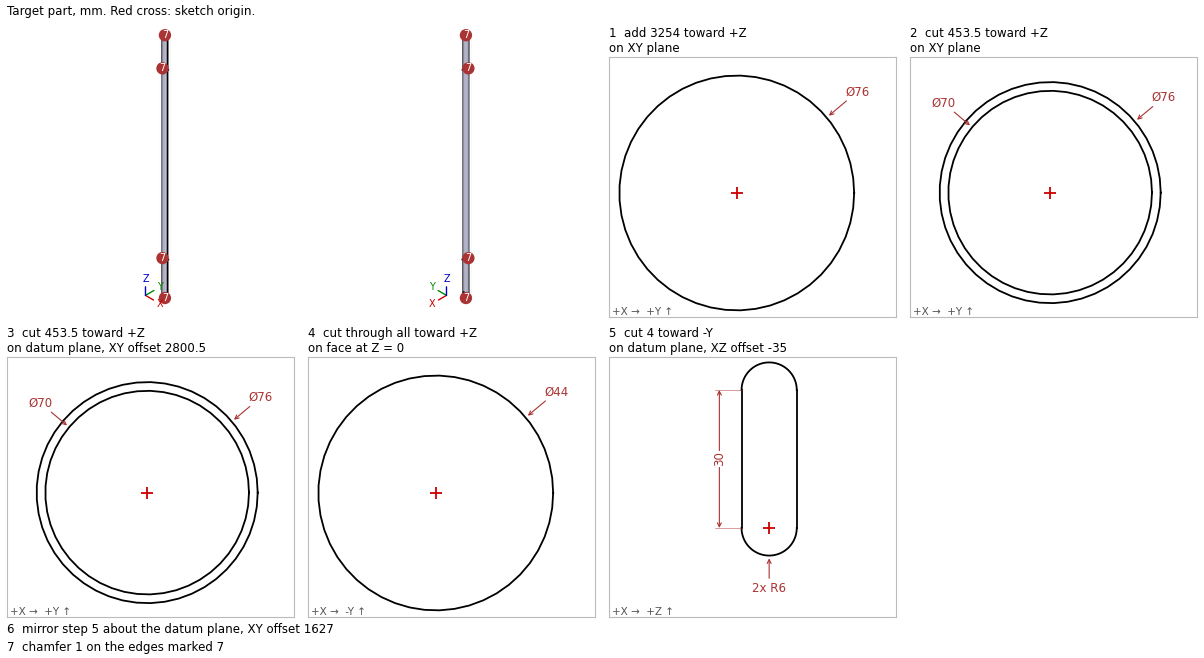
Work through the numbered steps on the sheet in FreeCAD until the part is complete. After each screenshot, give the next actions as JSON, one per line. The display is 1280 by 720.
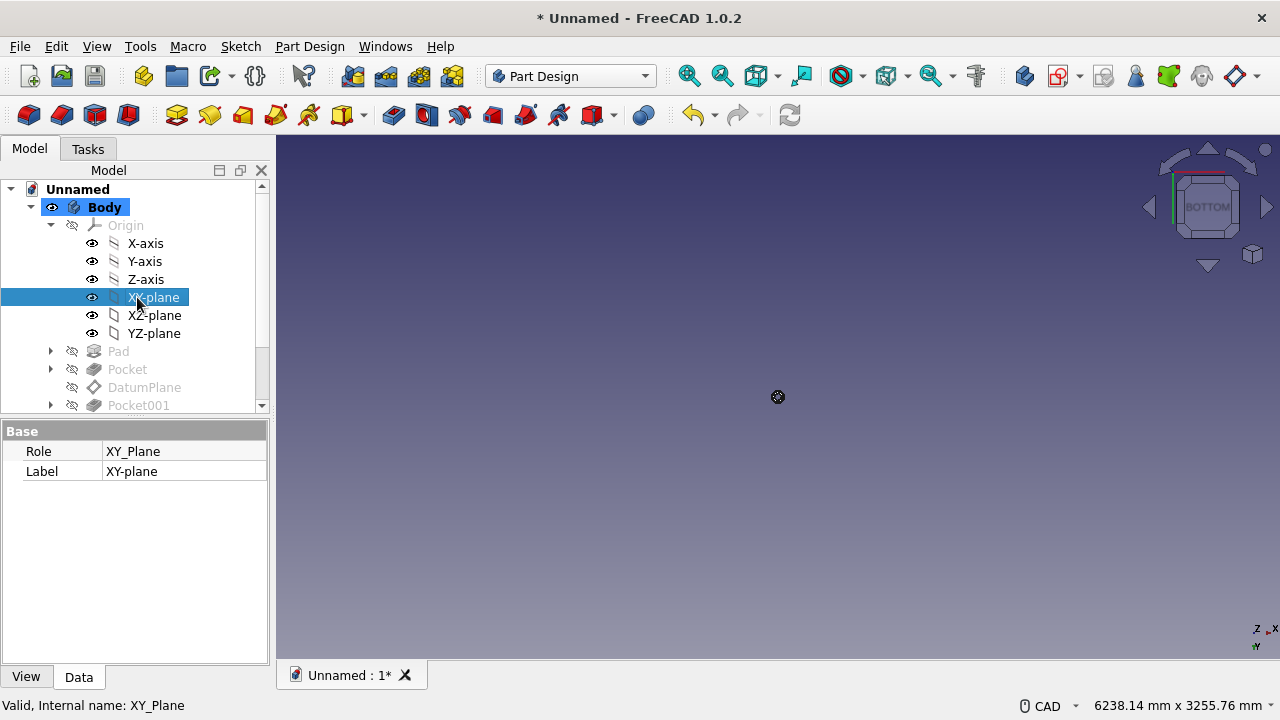
{"action": "left_click", "coordinate": [1234, 76]}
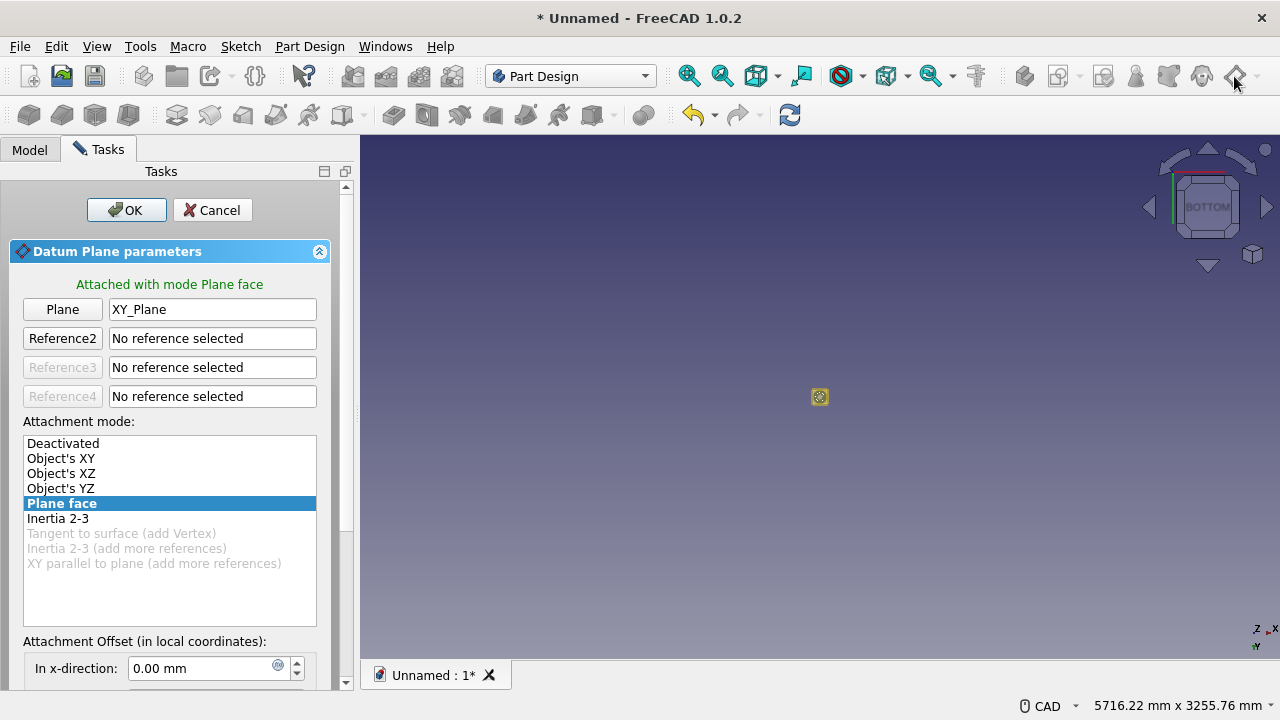
{"action": "scroll", "coordinate": [346, 436], "scroll_direction": "down", "scroll_amount": 2}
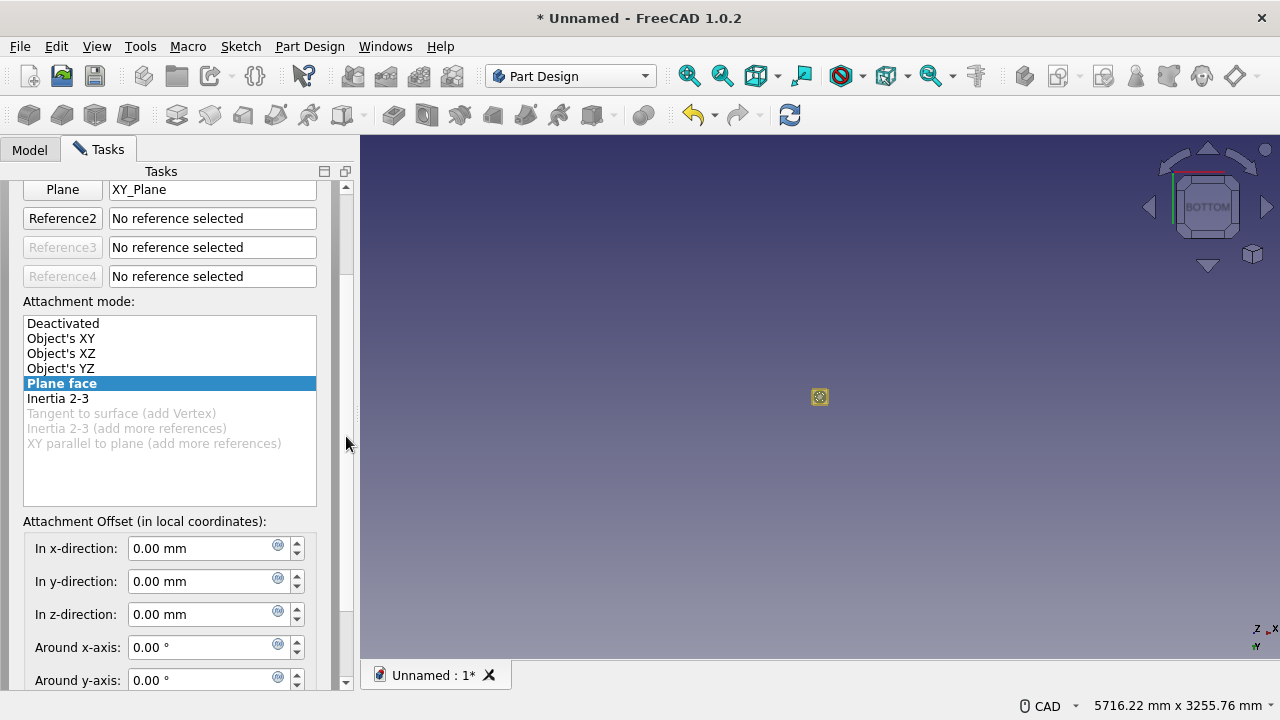
{"action": "triple_click", "coordinate": [210, 614]}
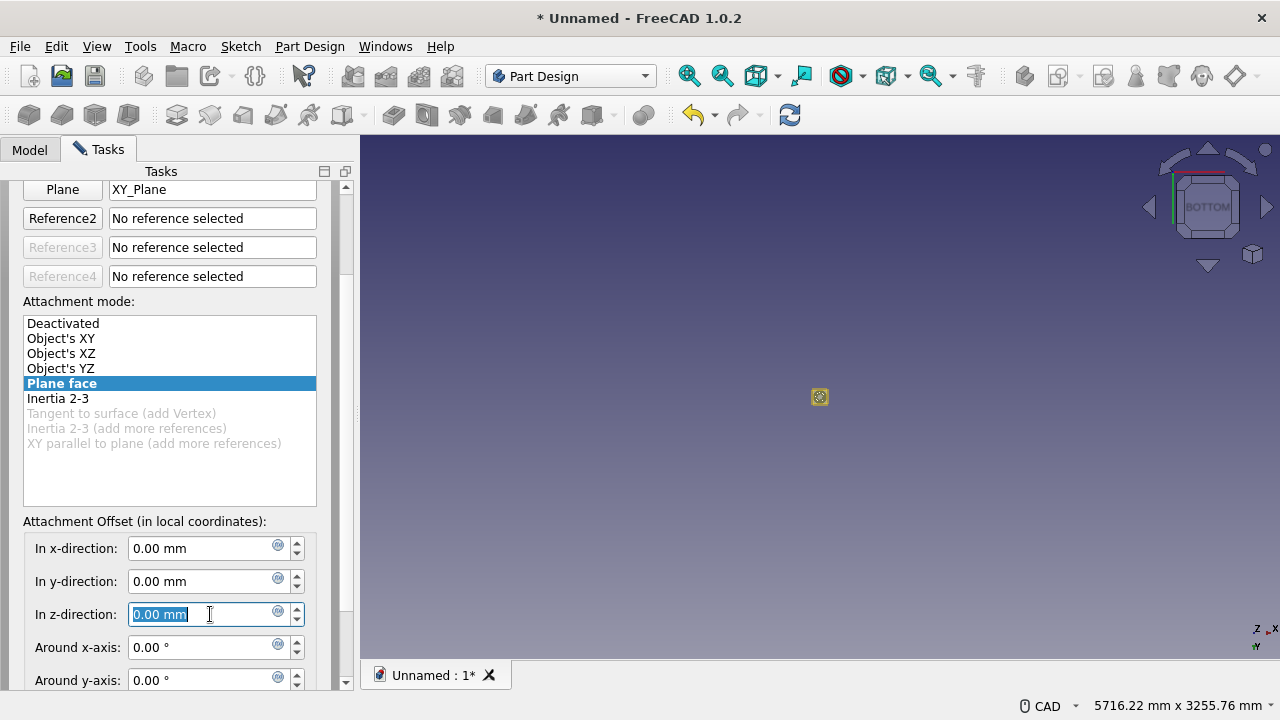
{"action": "type", "text": "1627"}
{"action": "key", "text": "Tab"}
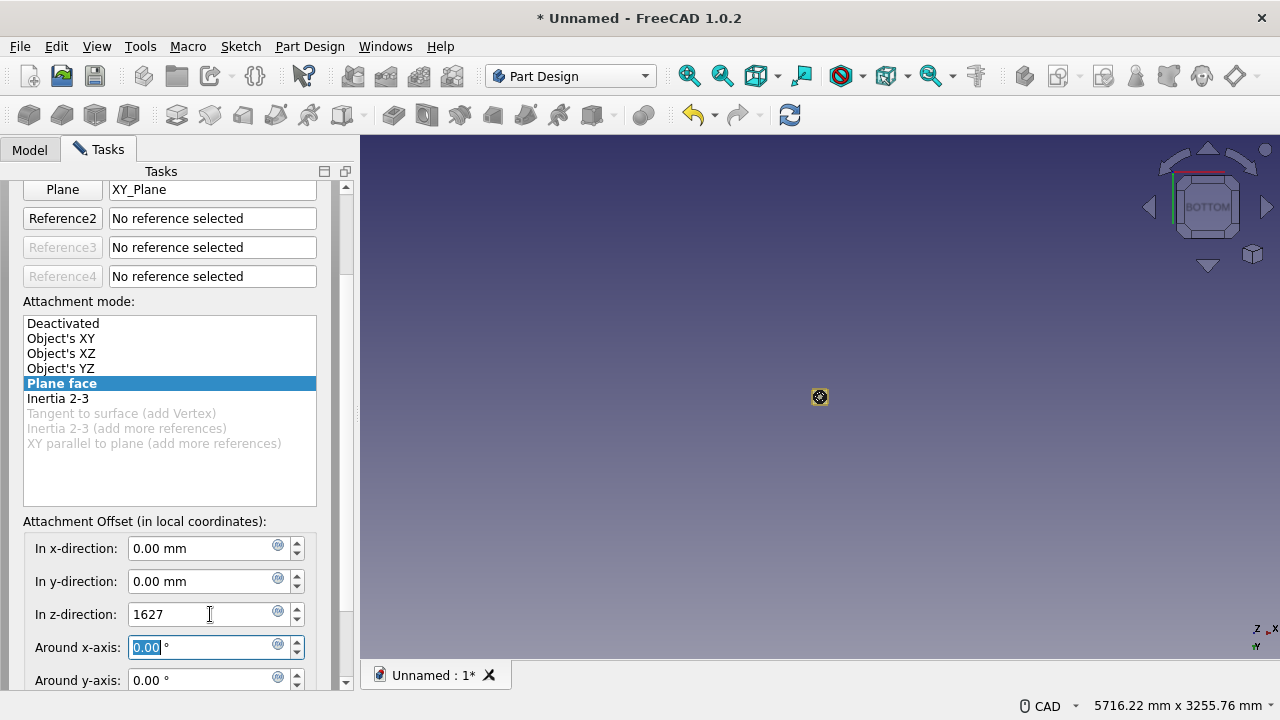
{"action": "scroll", "coordinate": [346, 436], "scroll_direction": "up", "scroll_amount": 3}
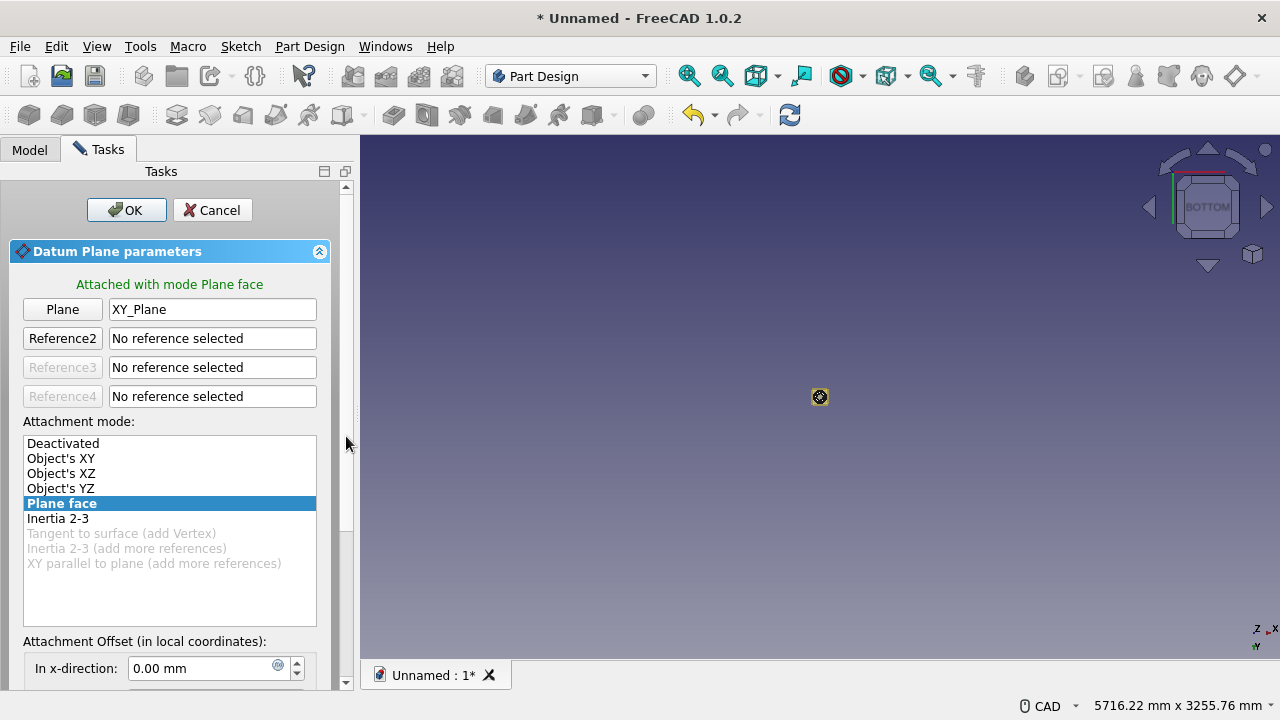
{"action": "left_click", "coordinate": [127, 210]}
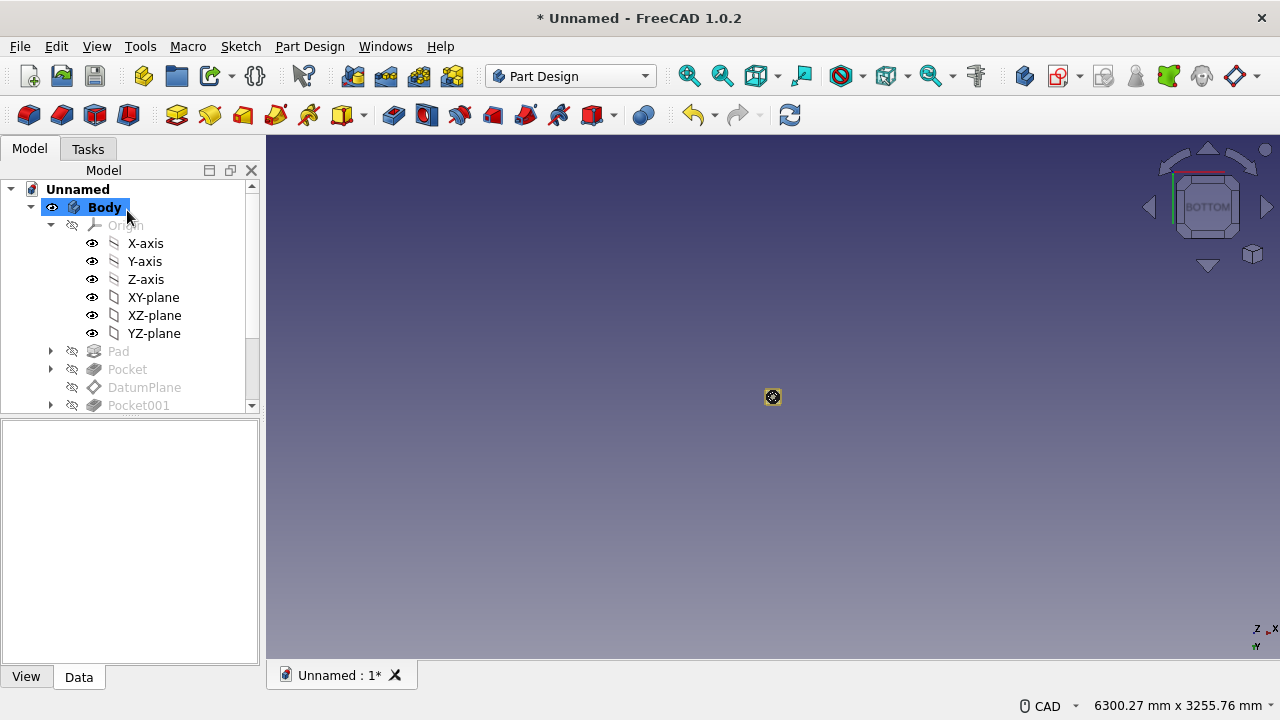
{"action": "scroll", "coordinate": [101, 293], "scroll_direction": "down", "scroll_amount": 3}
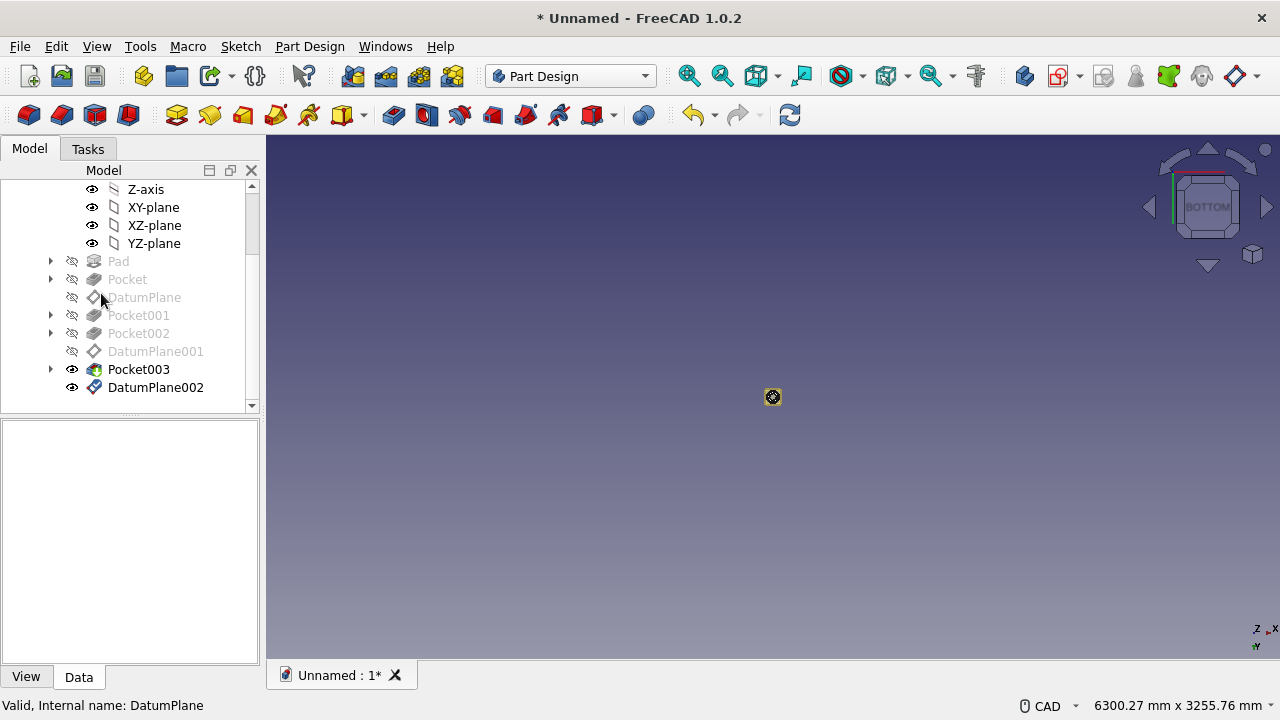
{"action": "left_click", "coordinate": [117, 369]}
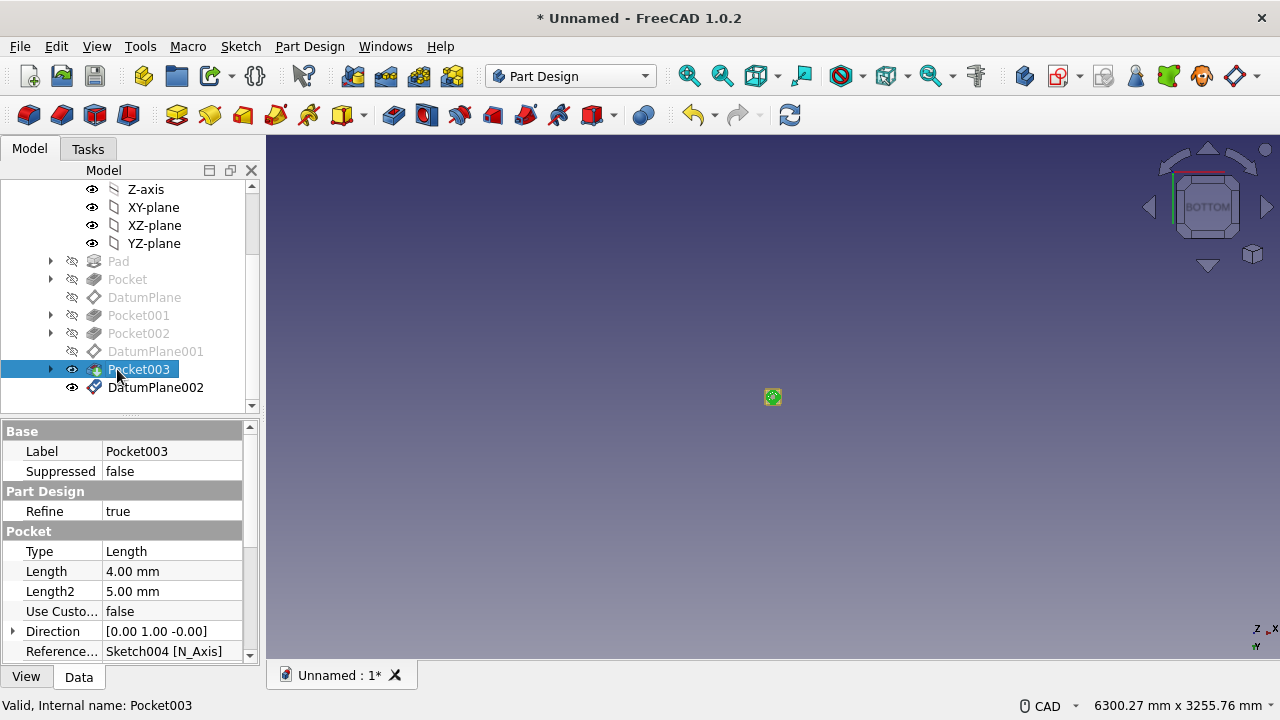
{"action": "left_click", "coordinate": [353, 76]}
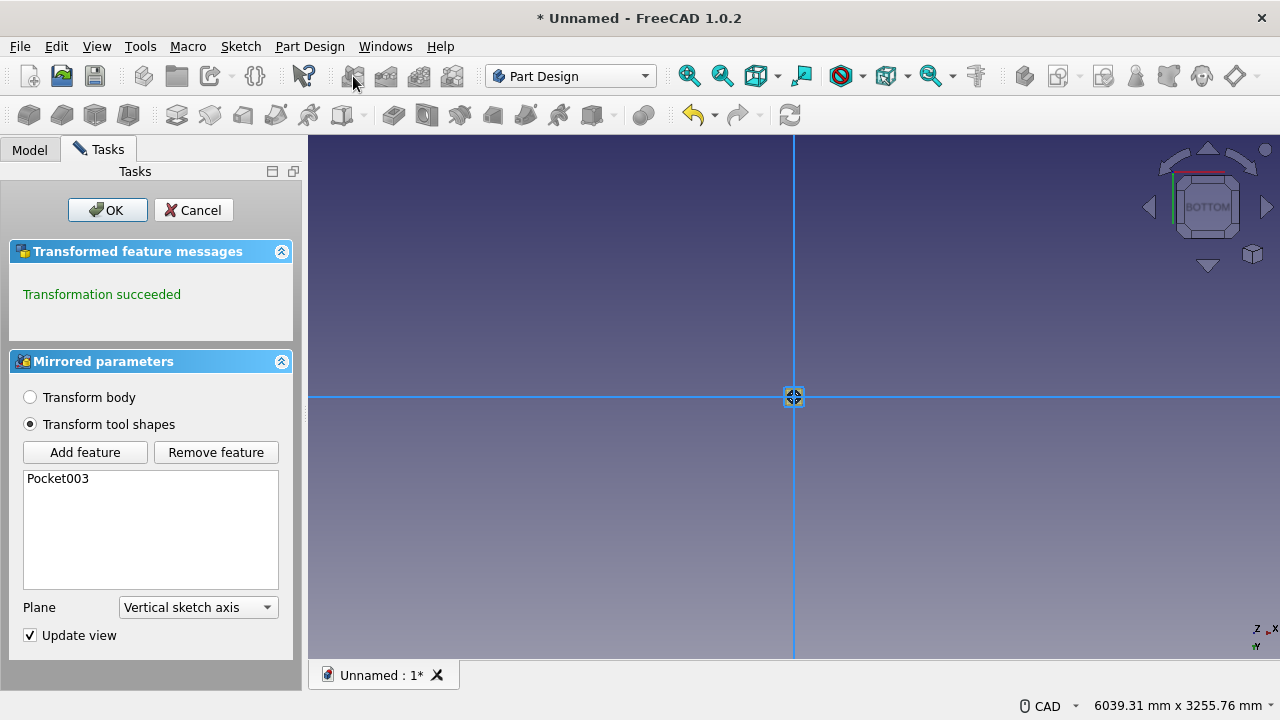
{"action": "left_click", "coordinate": [199, 608]}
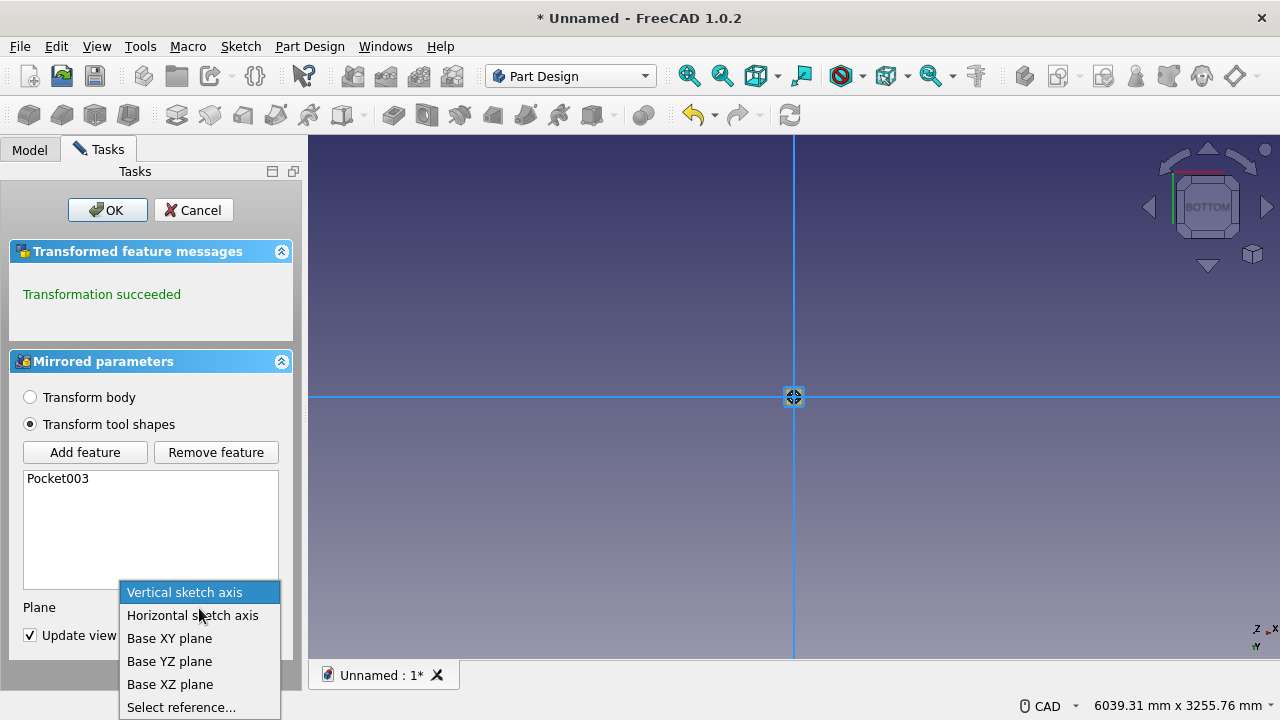
{"action": "left_click", "coordinate": [198, 708]}